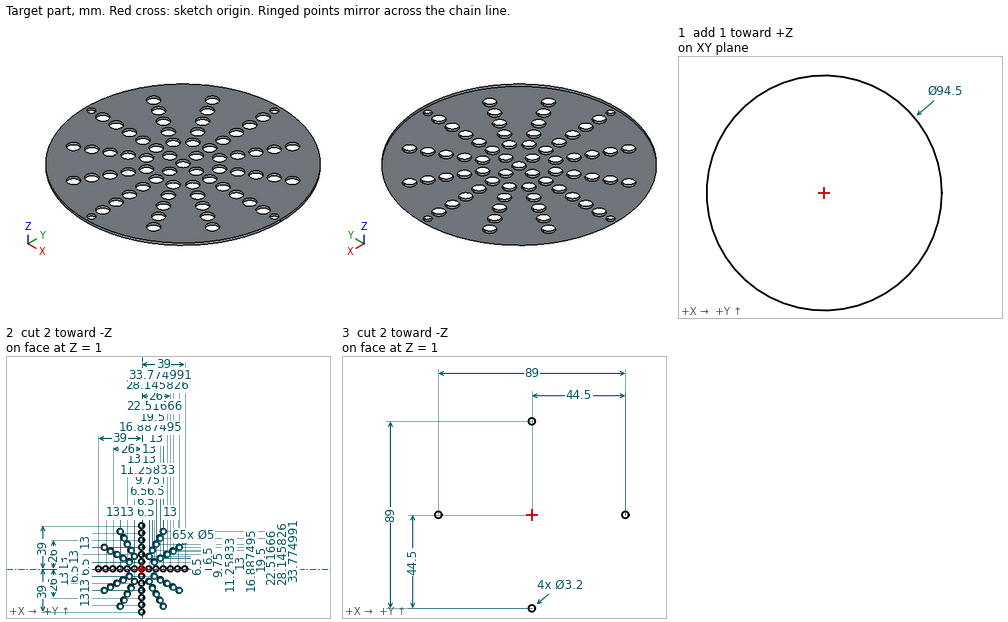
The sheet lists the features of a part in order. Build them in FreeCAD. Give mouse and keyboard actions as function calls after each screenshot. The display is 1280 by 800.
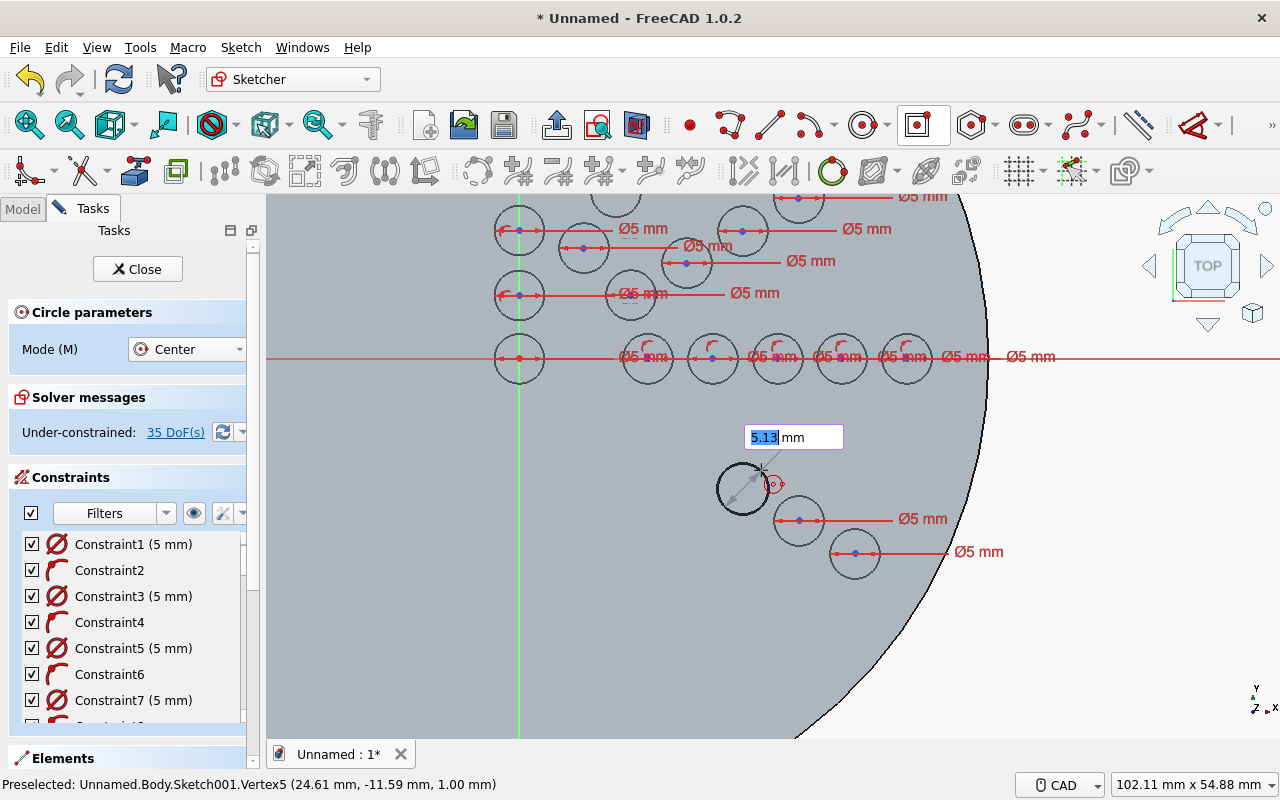
text(5)
key(Return)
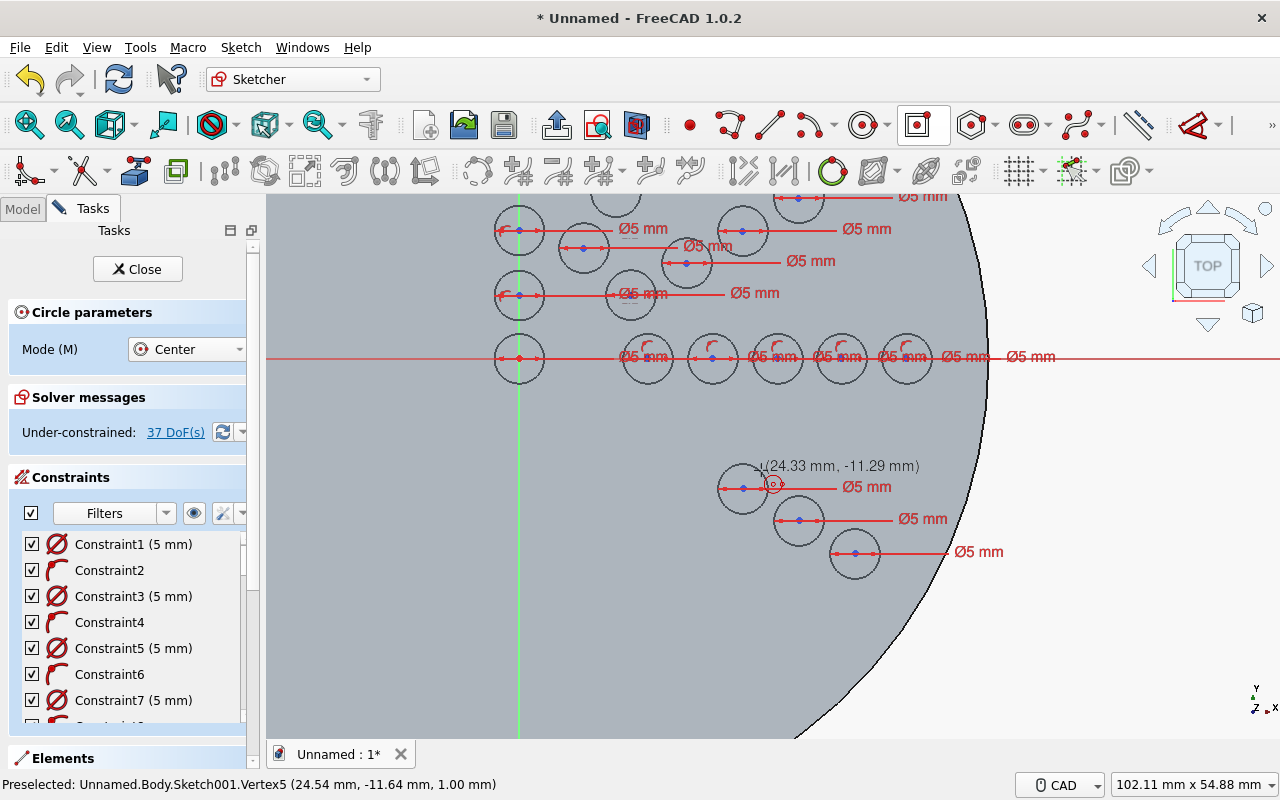
click(687, 456)
move(705, 438)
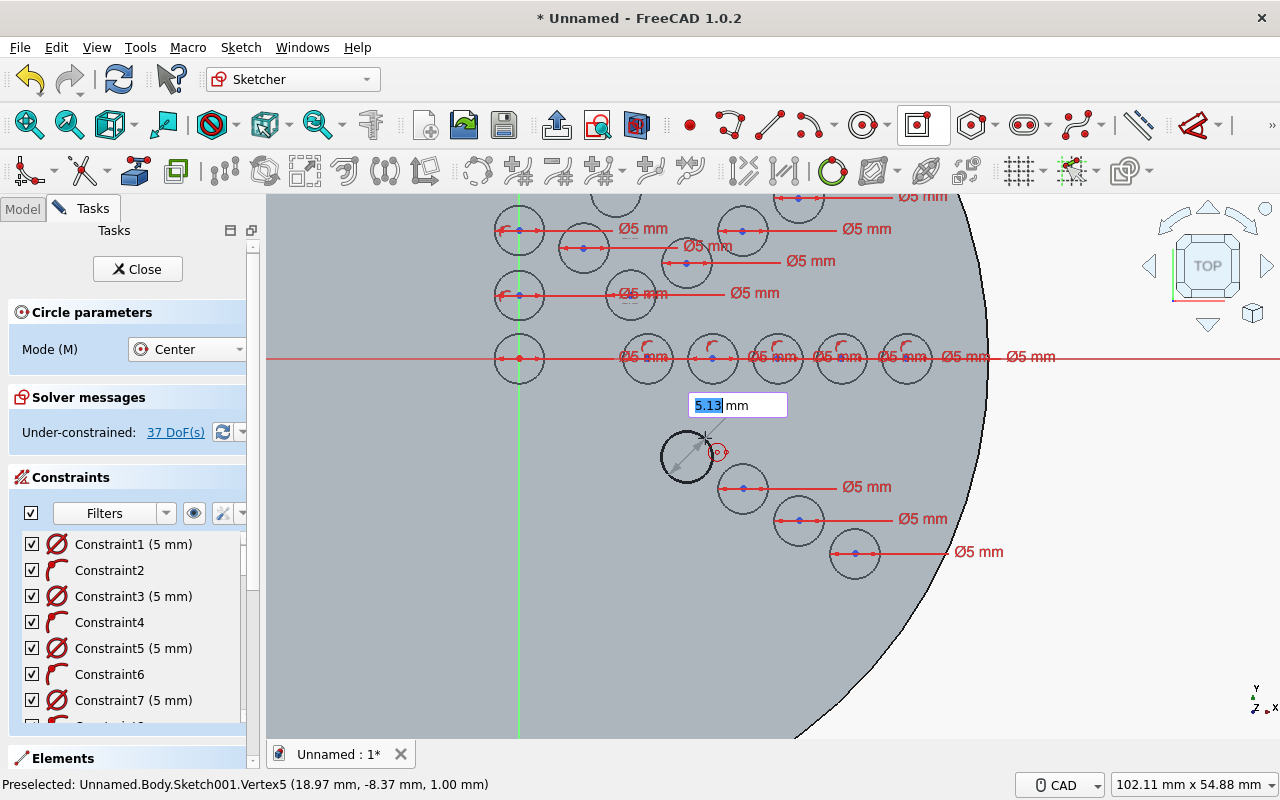
text(5)
key(Return)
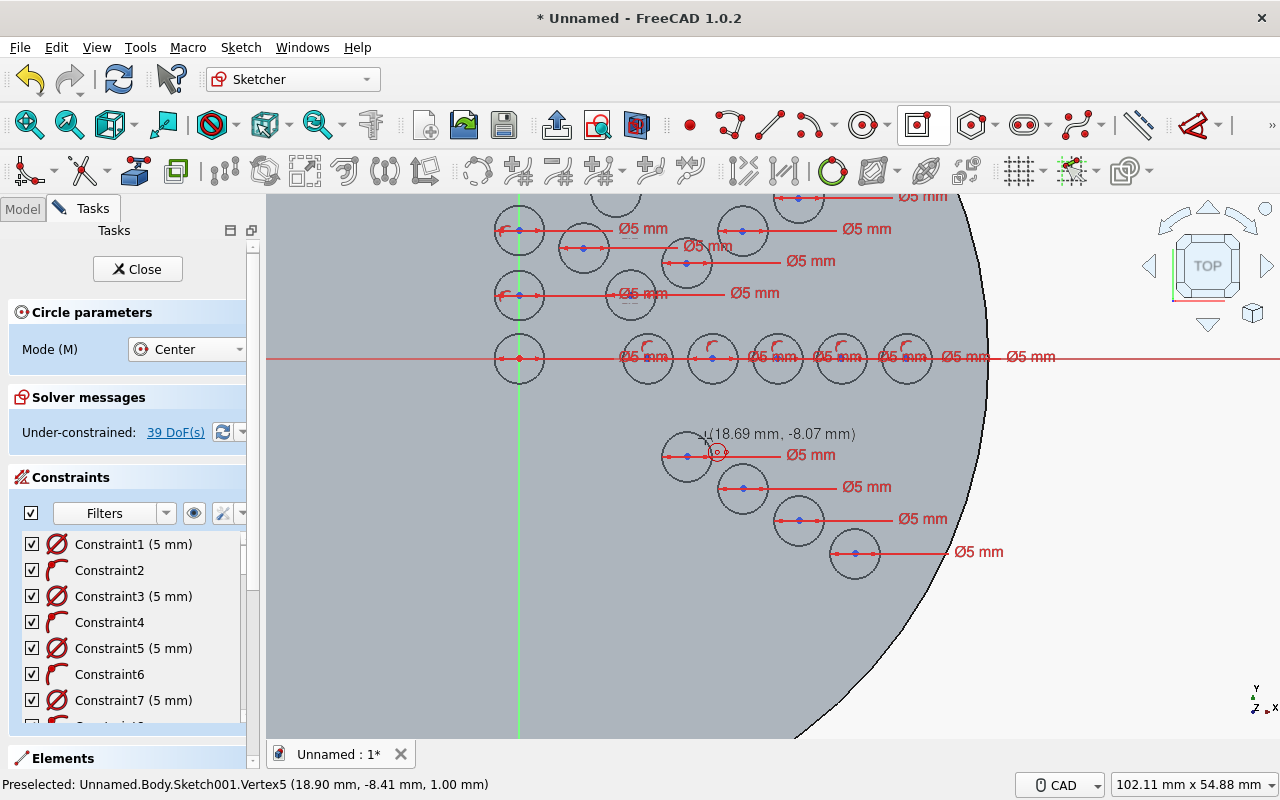
click(631, 423)
move(649, 406)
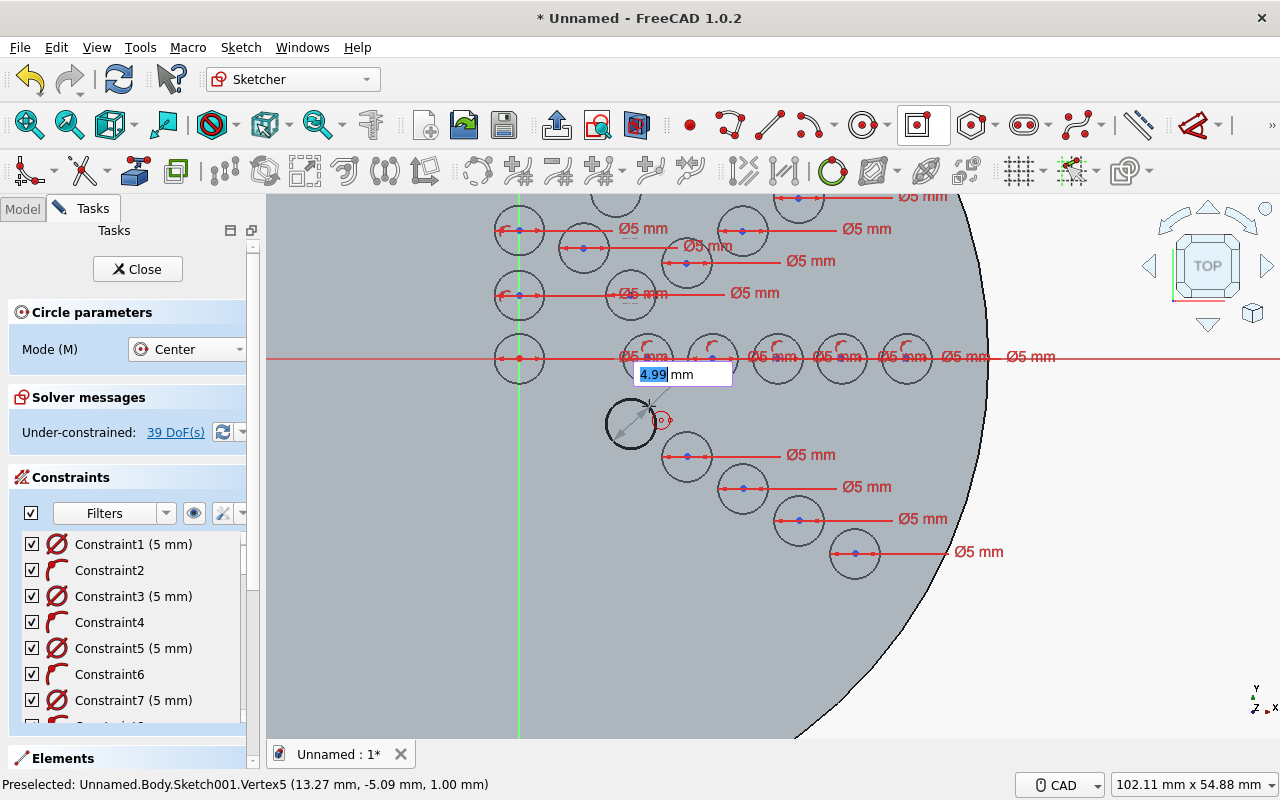
text(5)
key(Return)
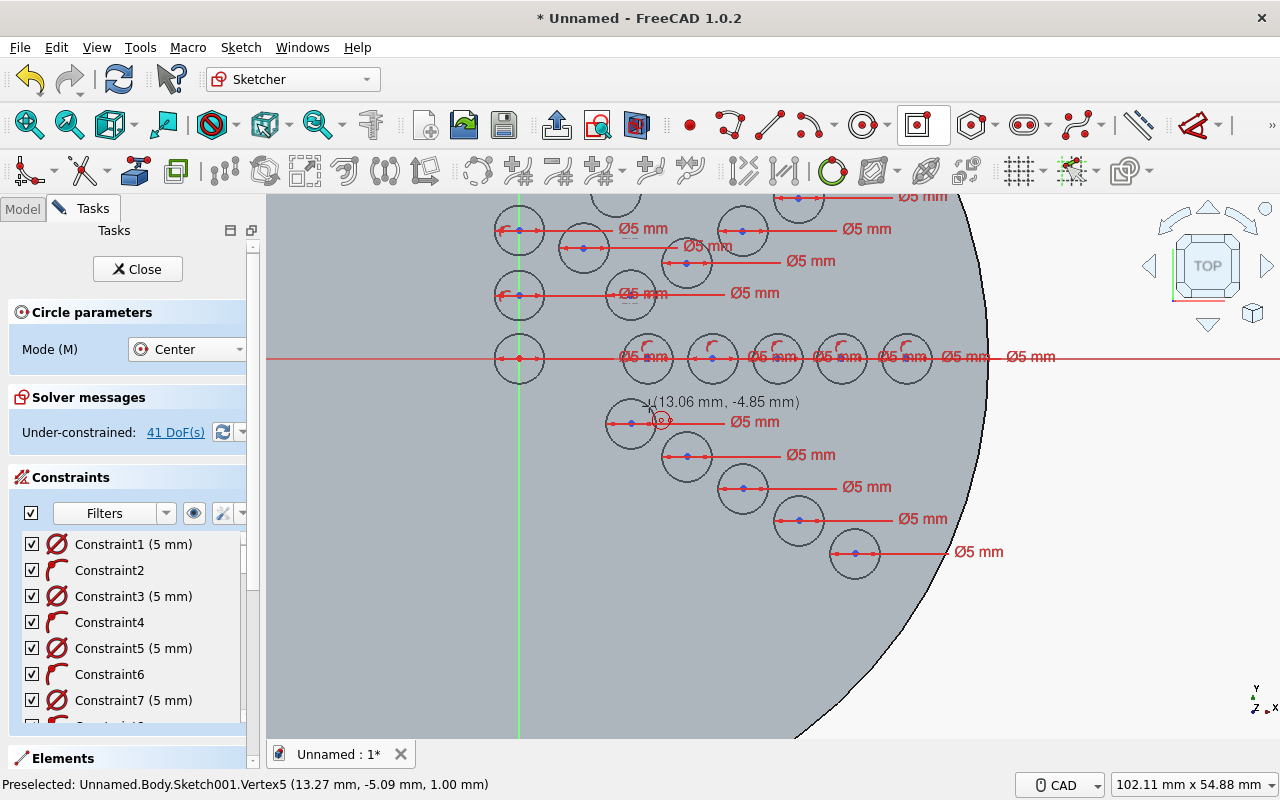
click(713, 694)
move(731, 677)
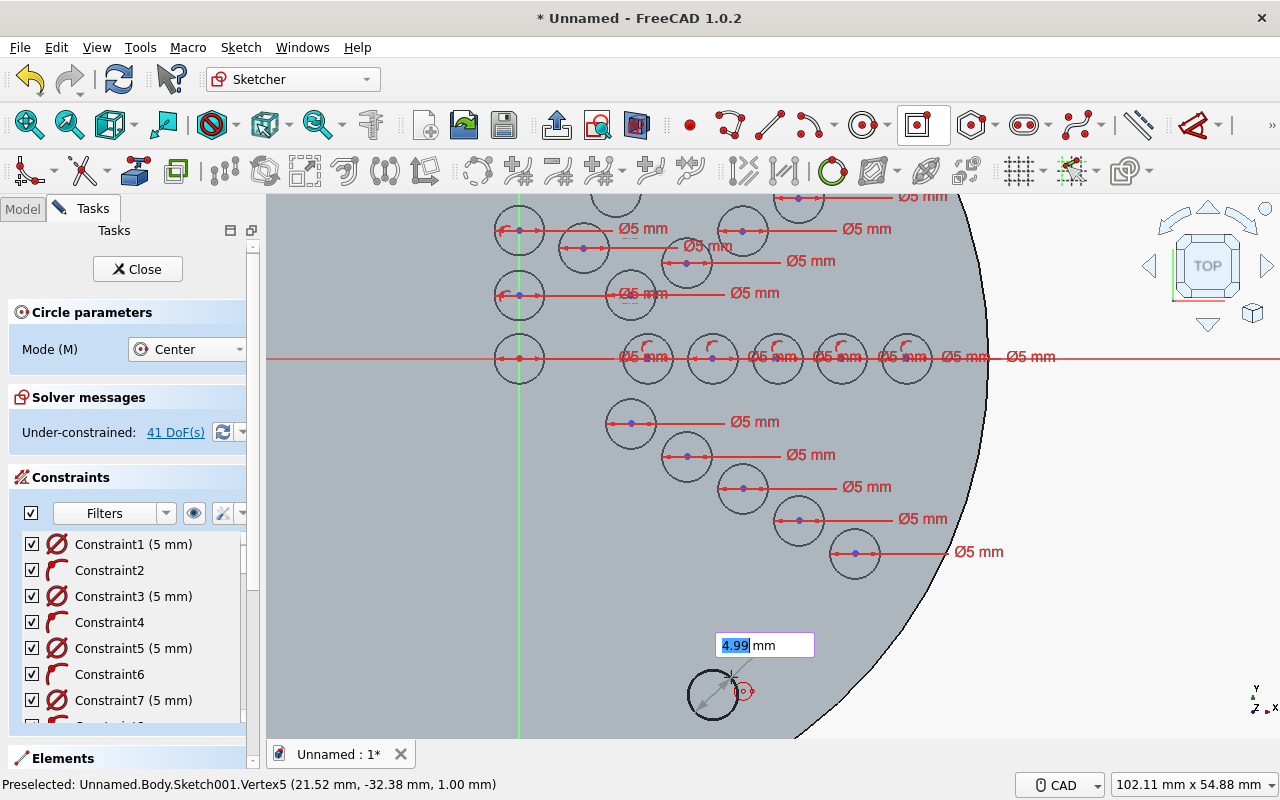
text(5)
key(Return)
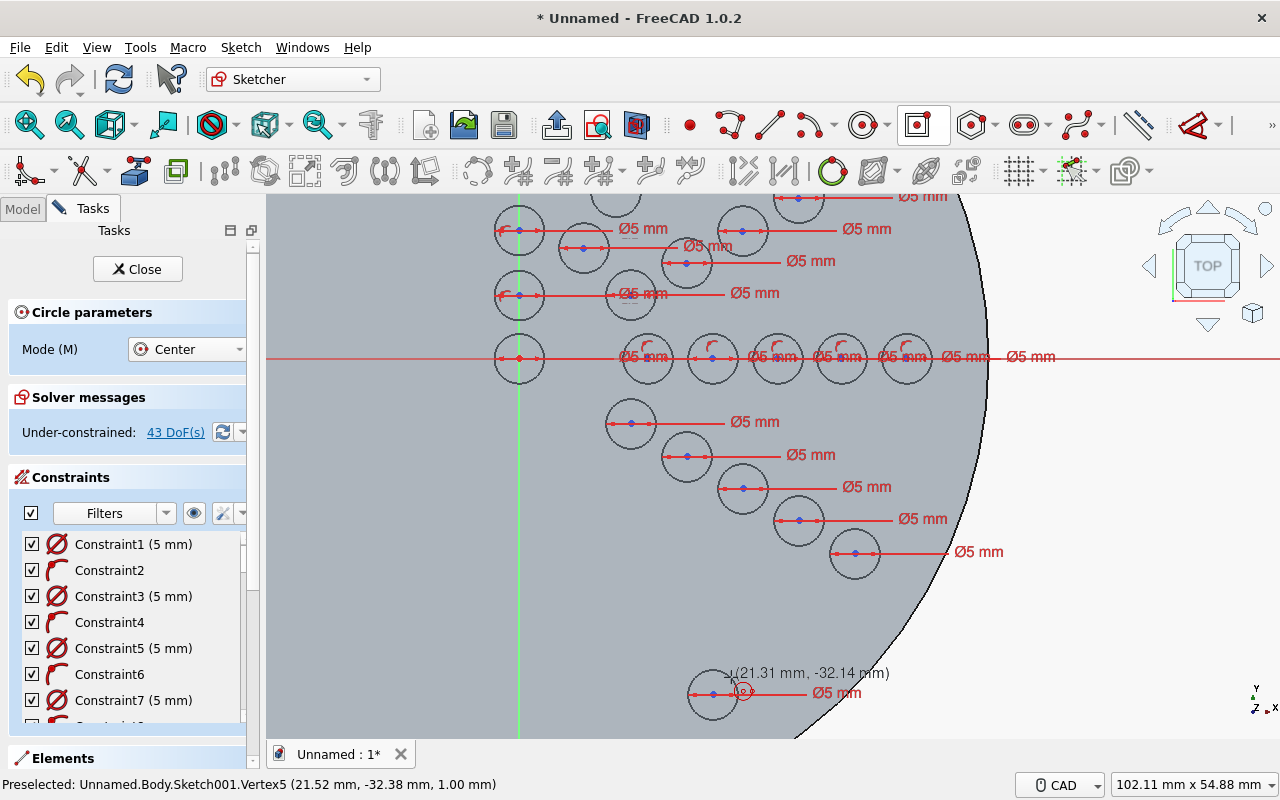
click(681, 638)
move(698, 621)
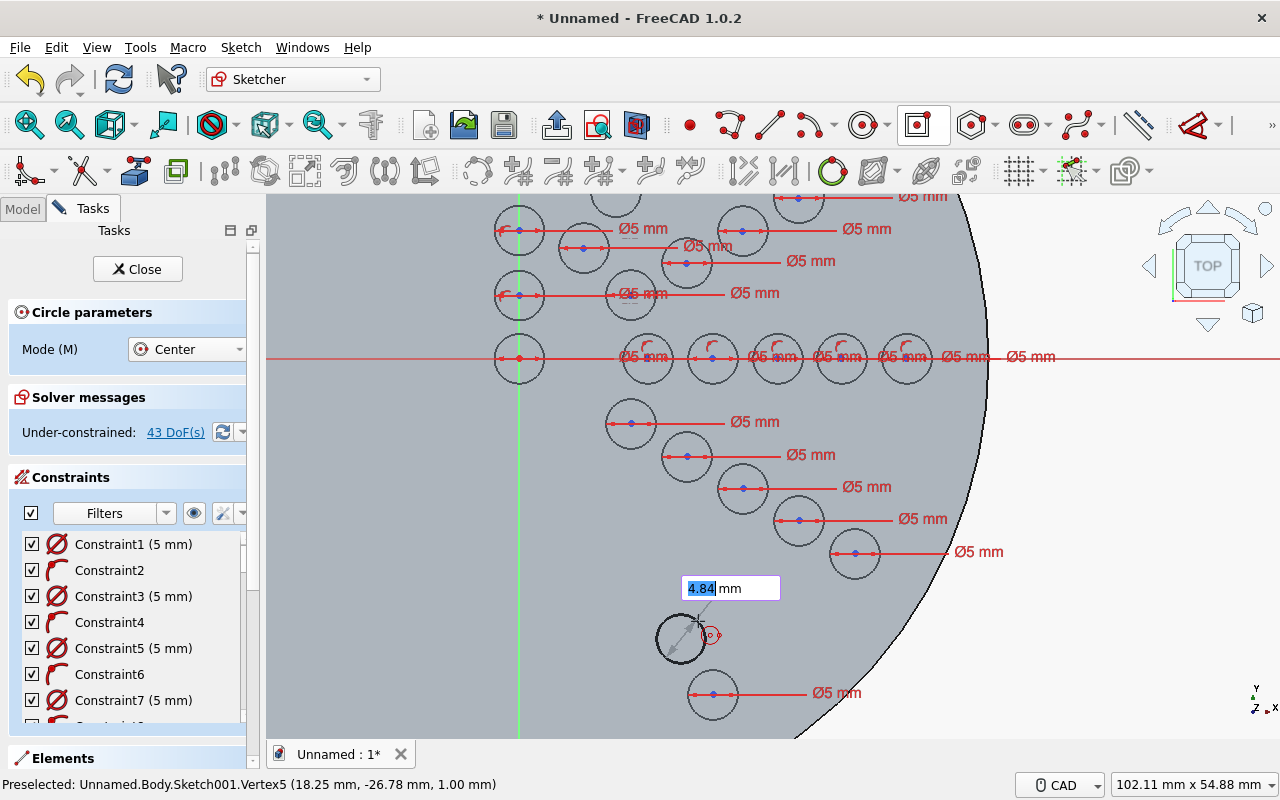
text(5)
key(Return)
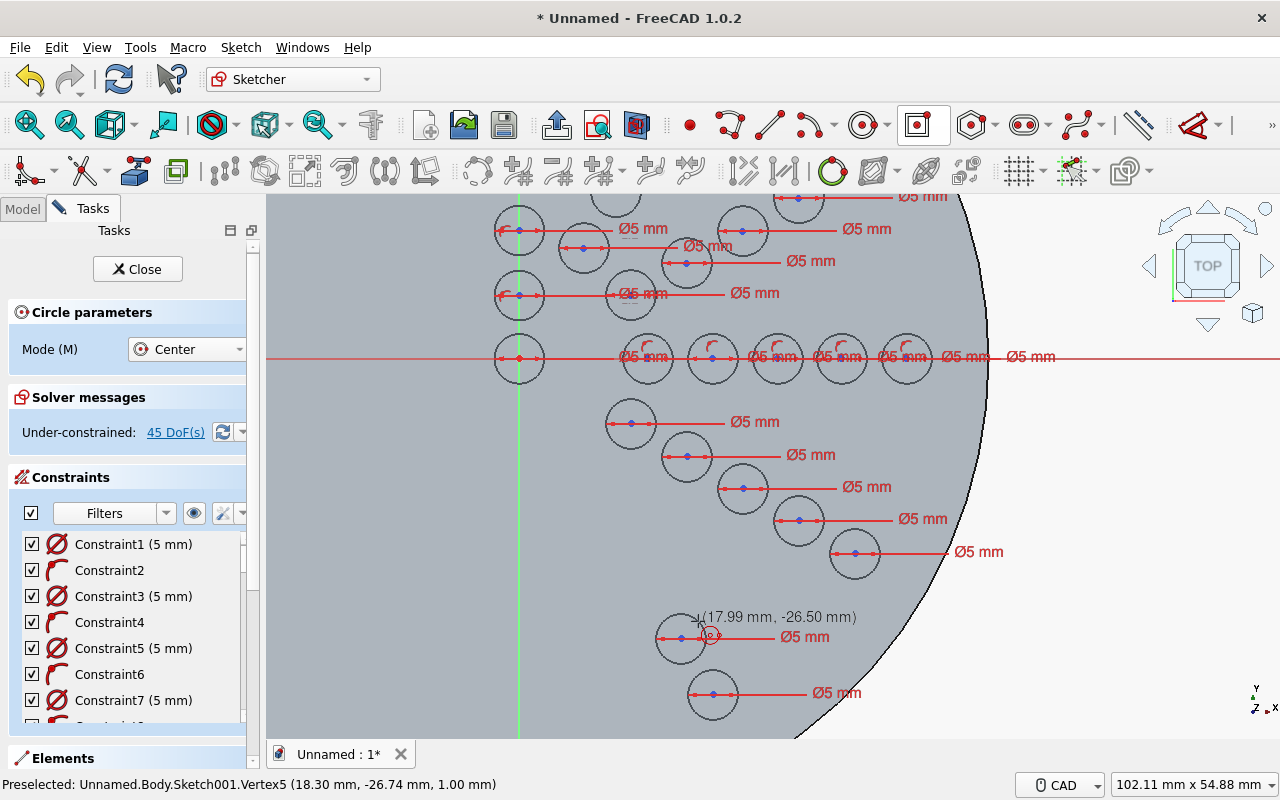
click(648, 582)
move(666, 565)